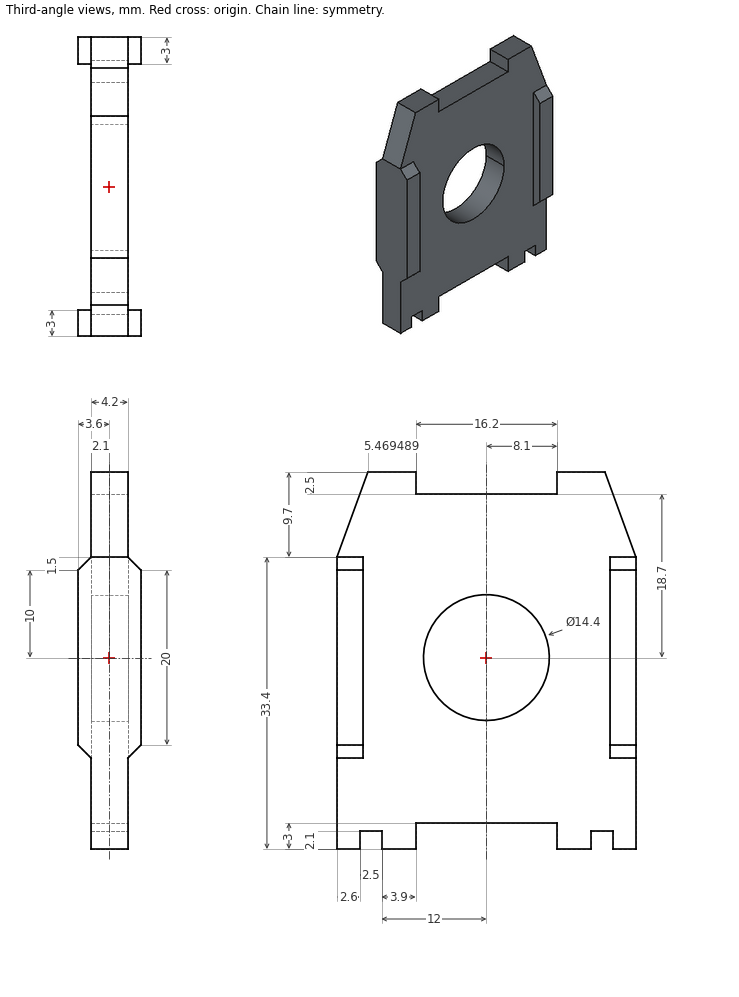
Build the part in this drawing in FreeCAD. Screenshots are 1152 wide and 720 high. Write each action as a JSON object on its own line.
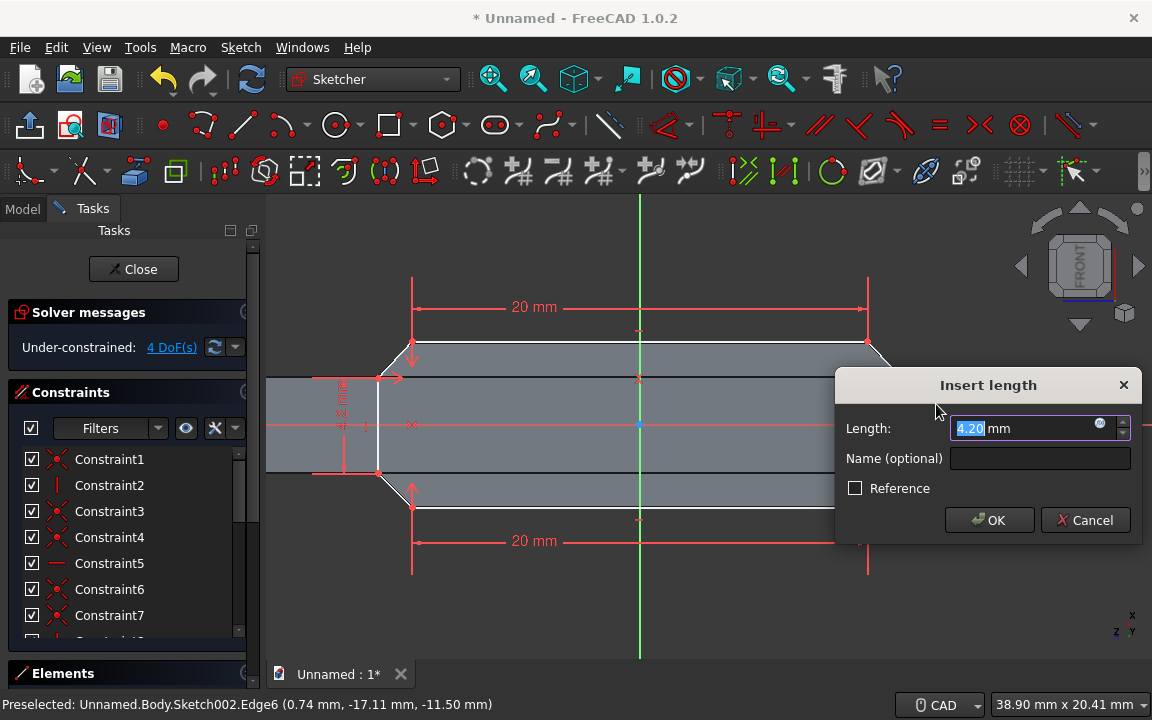
{"action": "type", "text": "4.2"}
{"action": "key", "text": "Return"}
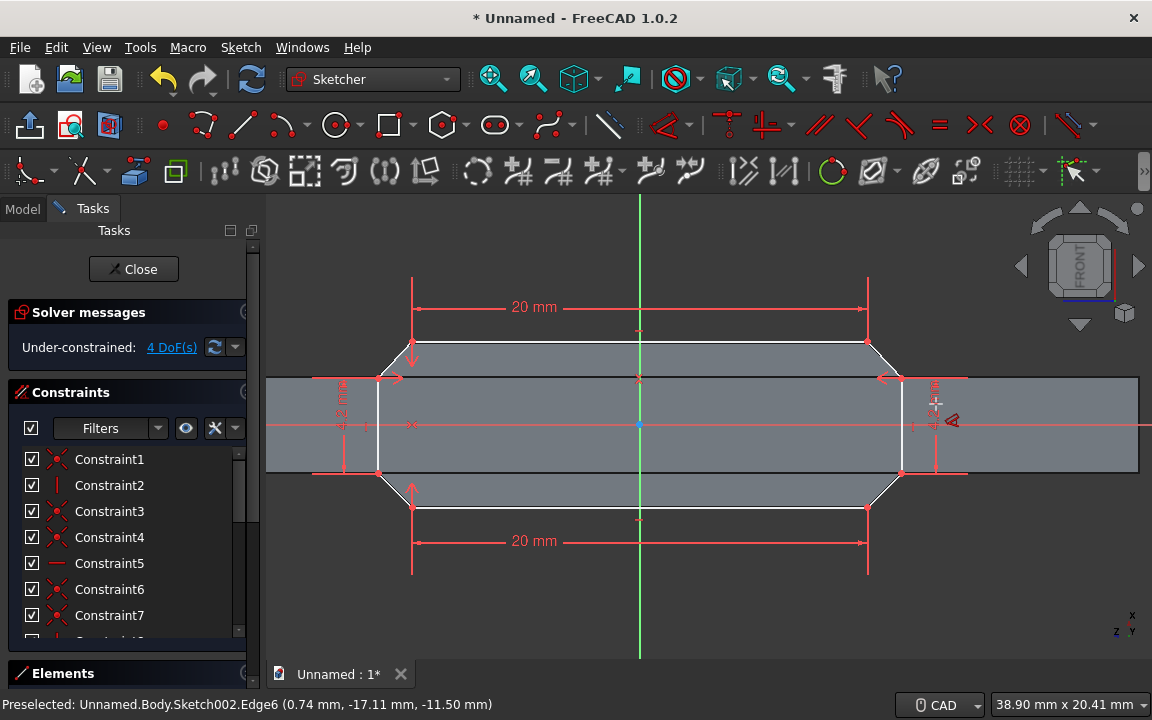
{"action": "left_click", "coordinate": [412, 508]}
{"action": "left_click", "coordinate": [446, 542]}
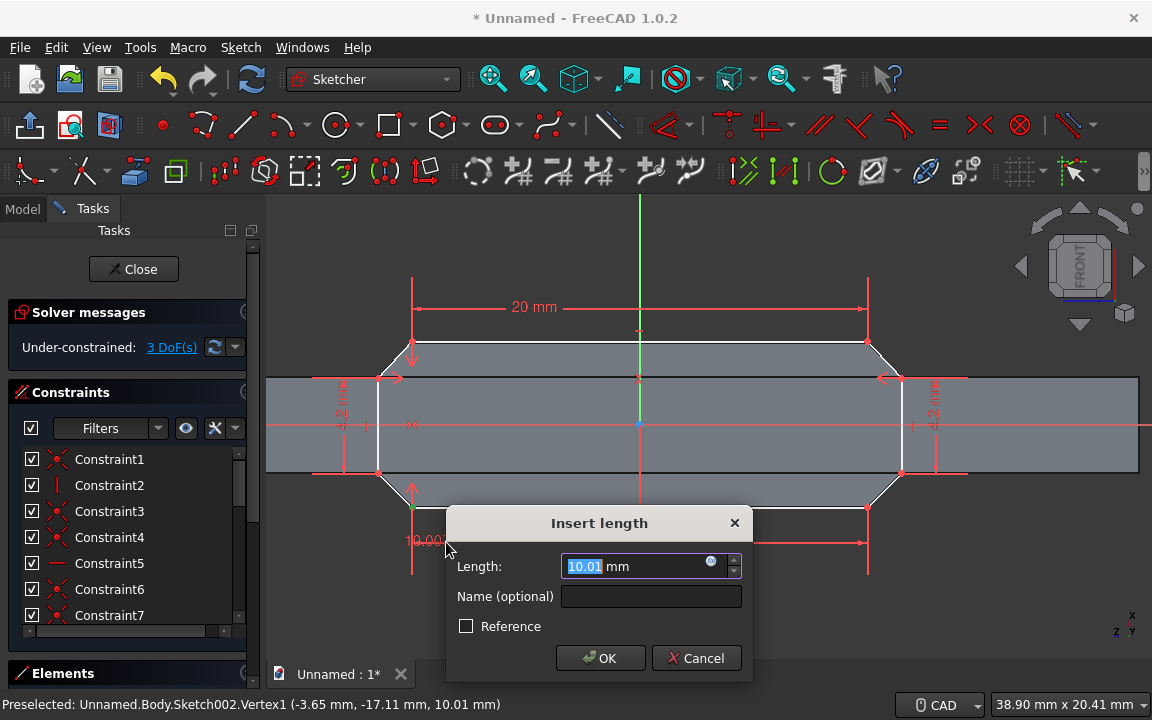
{"action": "type", "text": "10"}
{"action": "key", "text": "Return"}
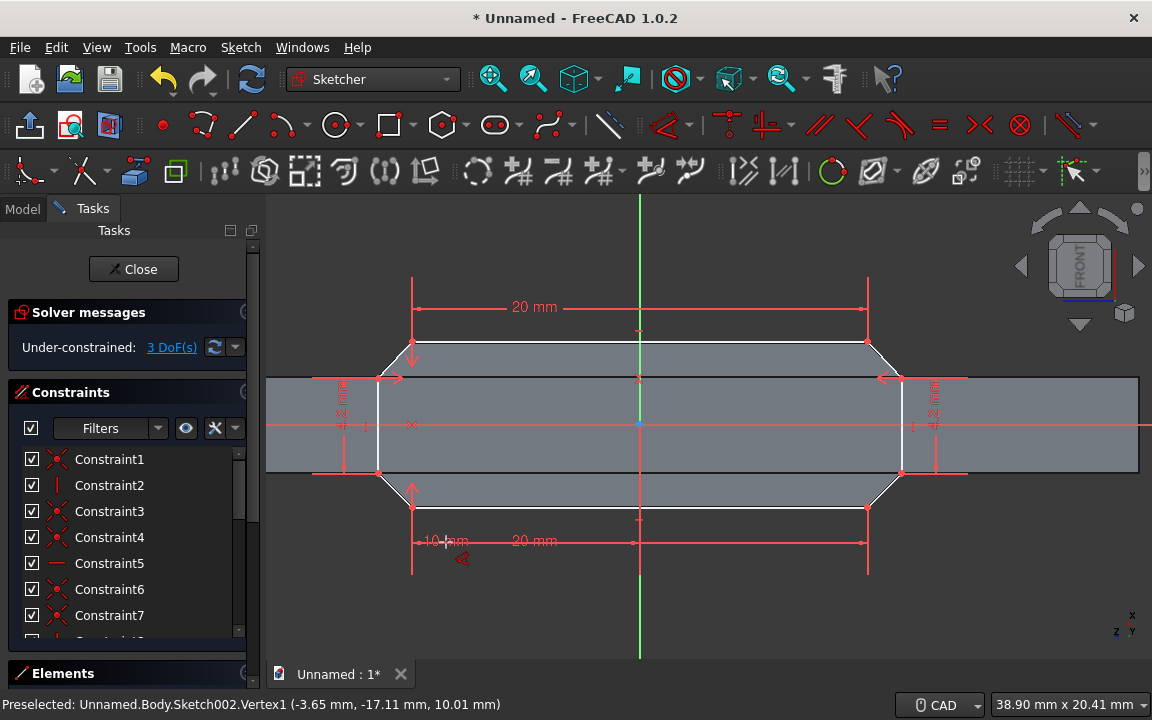
{"action": "left_click", "coordinate": [412, 508]}
{"action": "left_click", "coordinate": [378, 495]}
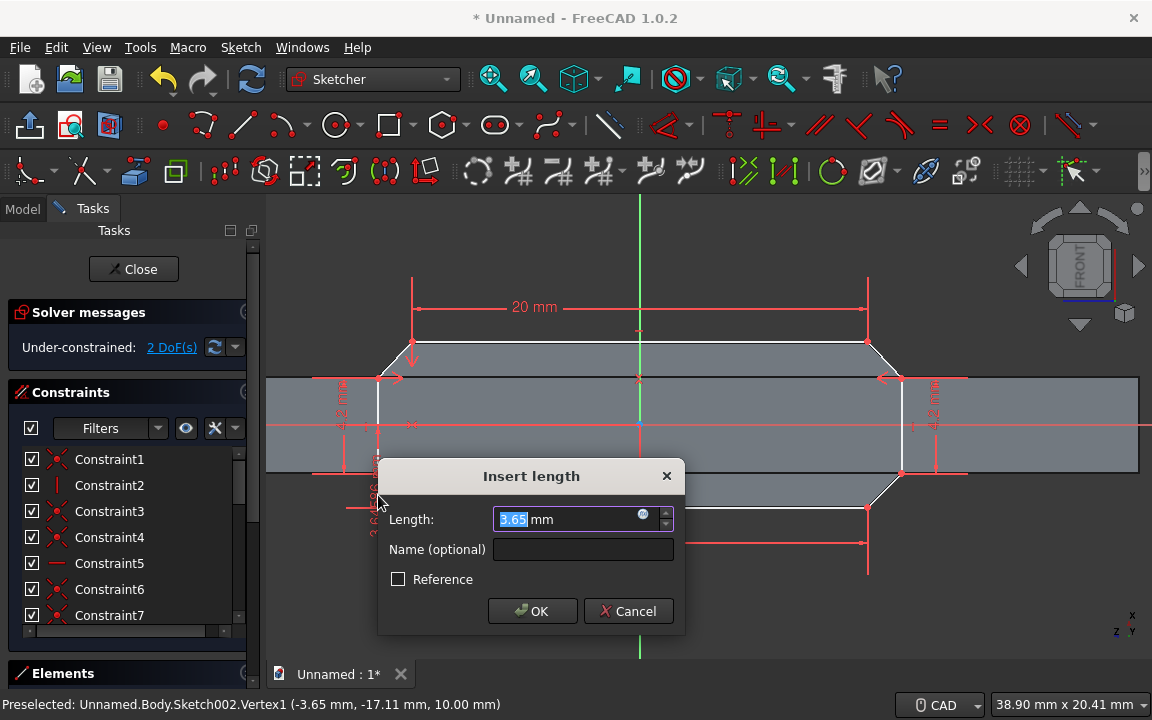
{"action": "type", "text": "3.6"}
{"action": "key", "text": "Return"}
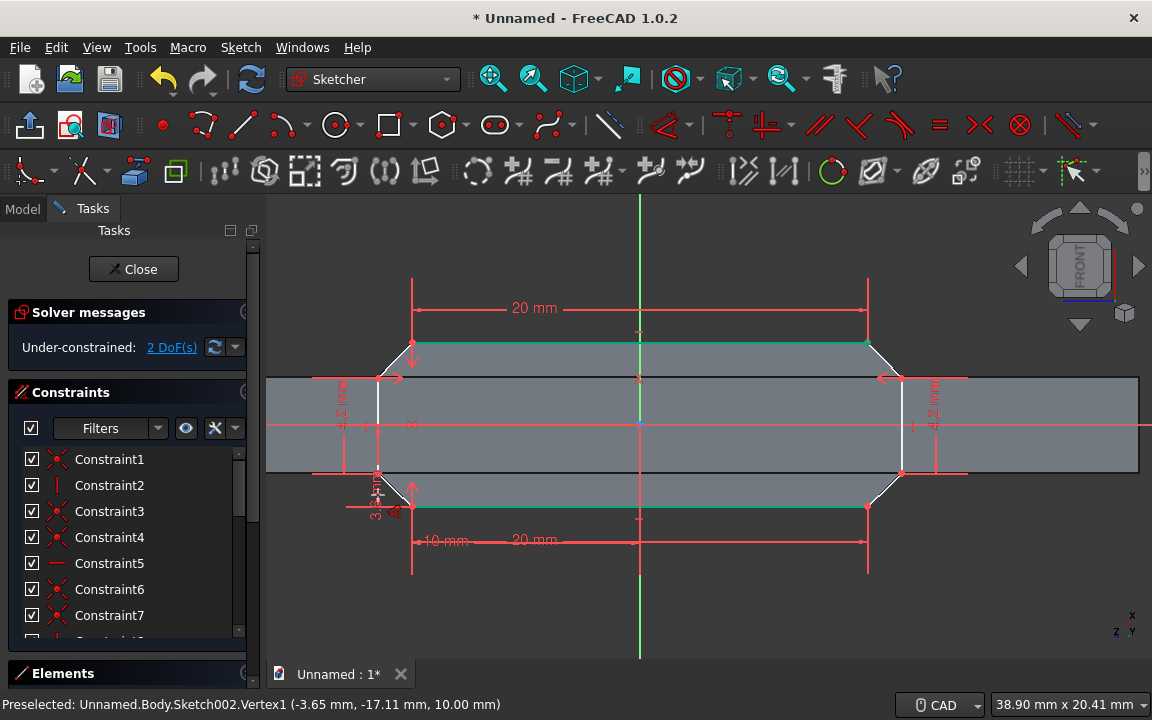
{"action": "left_click", "coordinate": [378, 474]}
{"action": "left_click", "coordinate": [344, 449]}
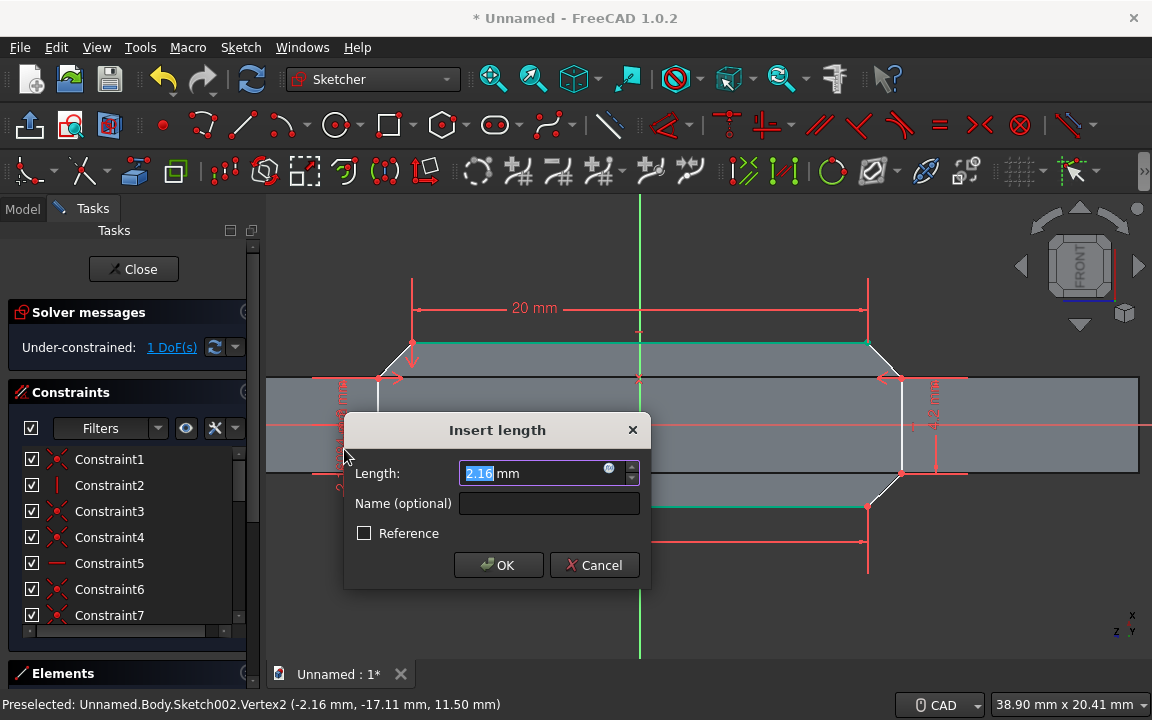
{"action": "type", "text": "2.1"}
{"action": "key", "text": "Return"}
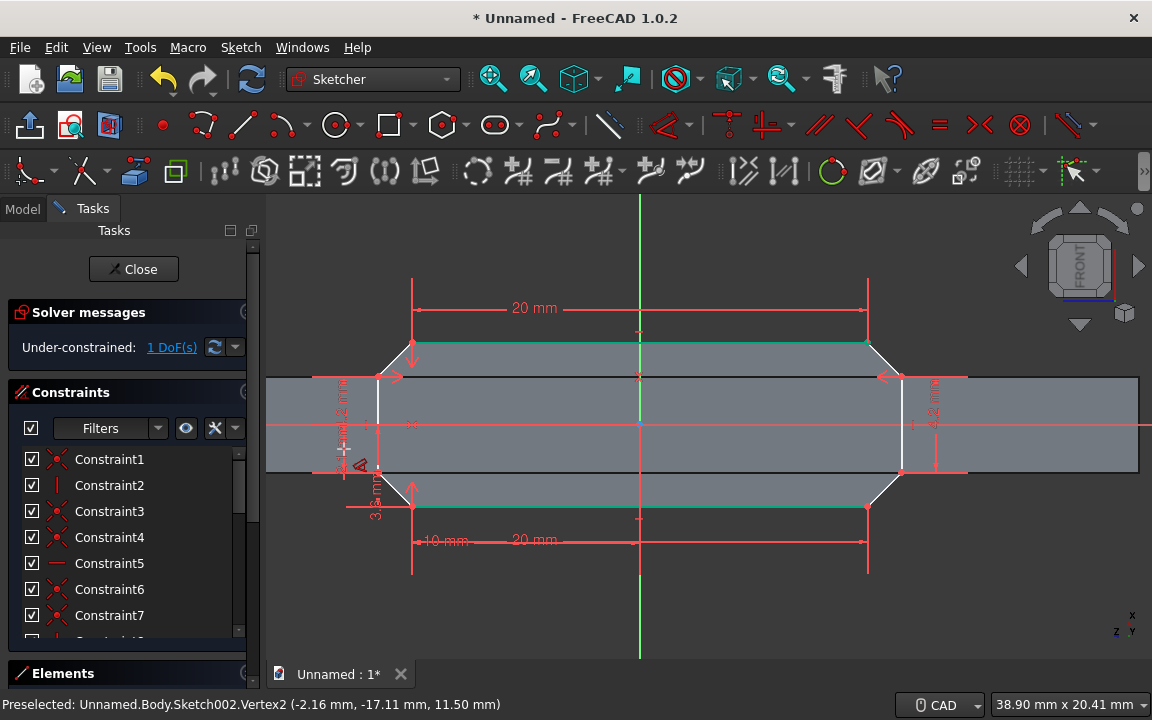
{"action": "left_click", "coordinate": [402, 497]}
{"action": "left_click", "coordinate": [395, 565]}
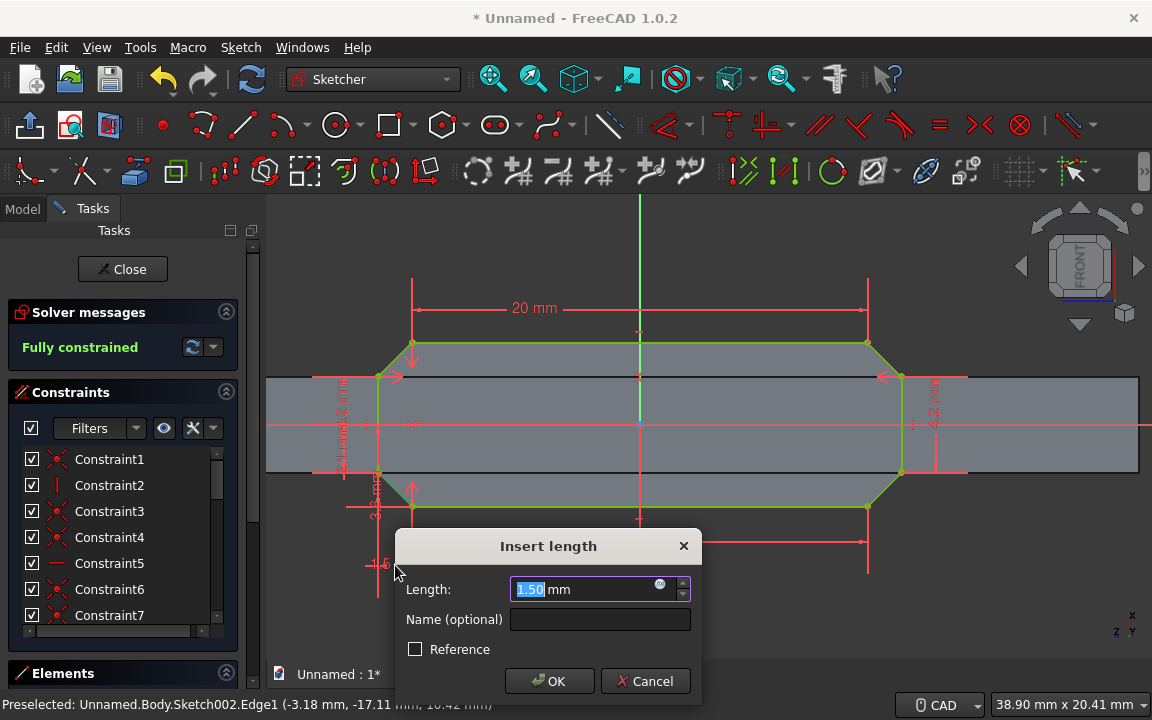
{"action": "type", "text": "1.5"}
{"action": "key", "text": "Return"}
{"action": "key", "text": "Escape"}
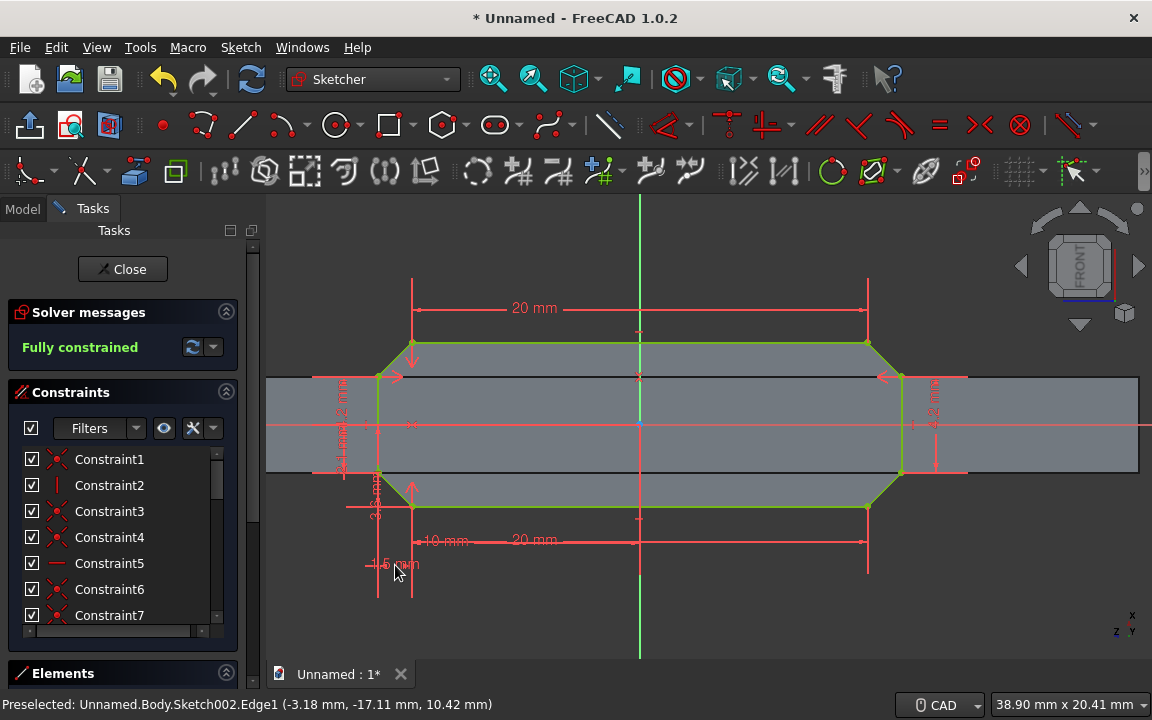
{"action": "left_click", "coordinate": [123, 269]}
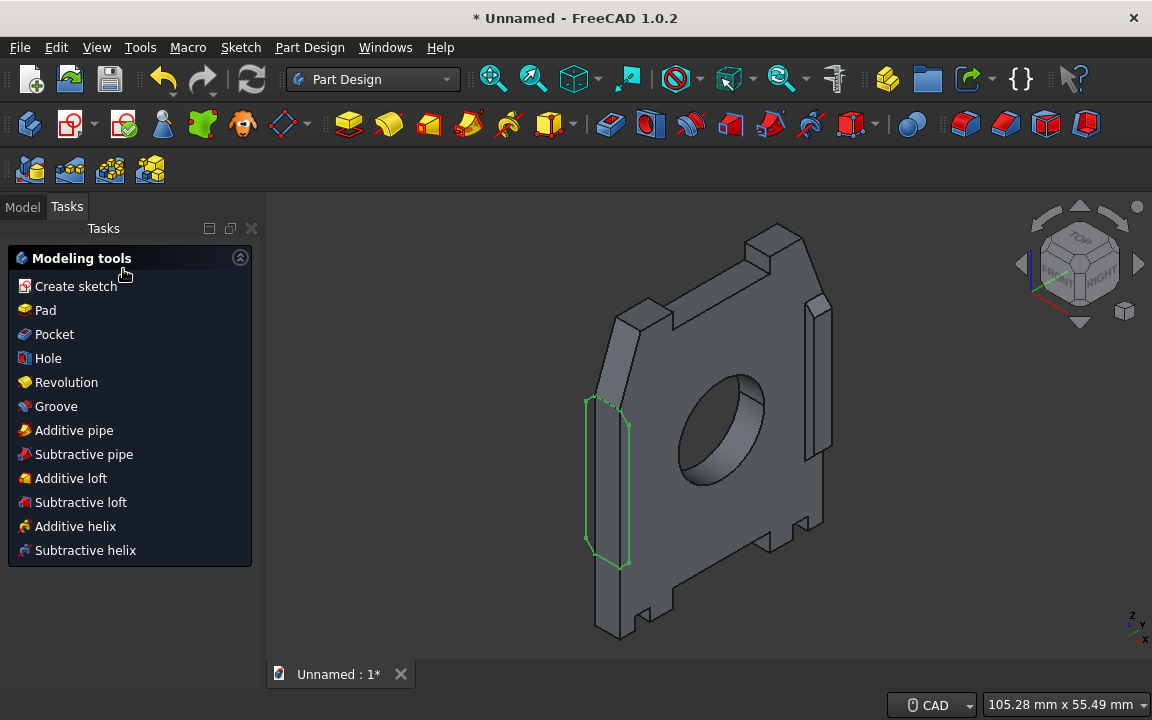
{"action": "left_click", "coordinate": [350, 124]}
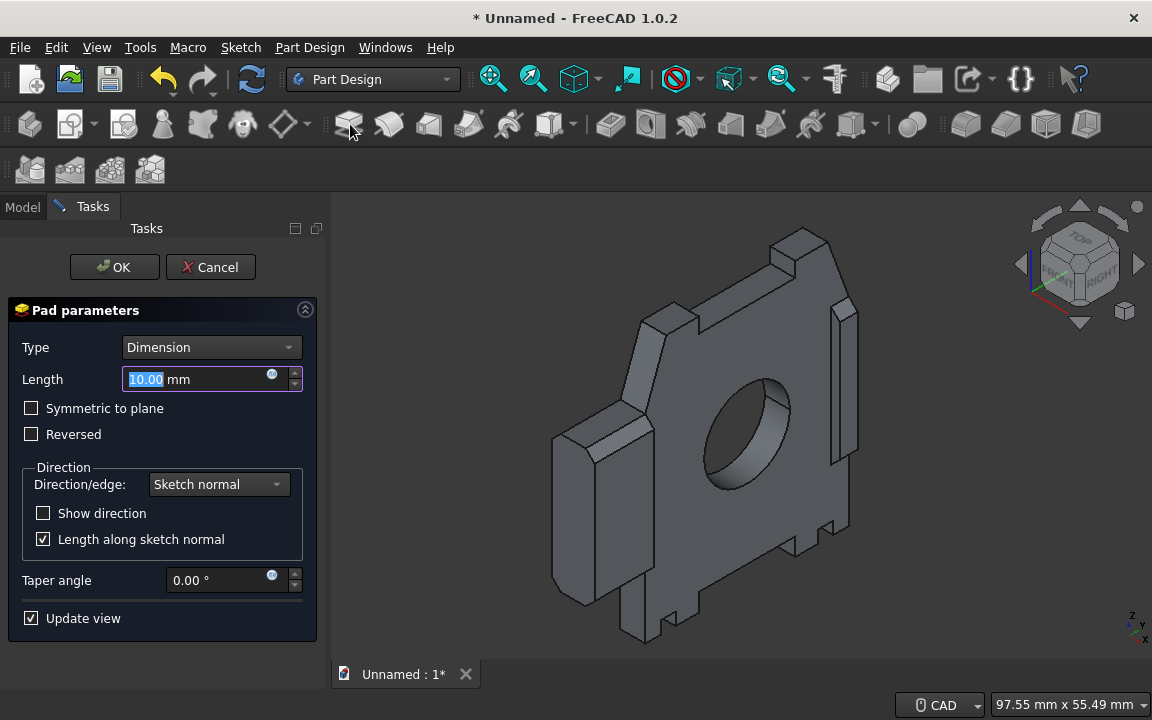
{"action": "type", "text": "3"}
{"action": "key", "text": "Tab"}